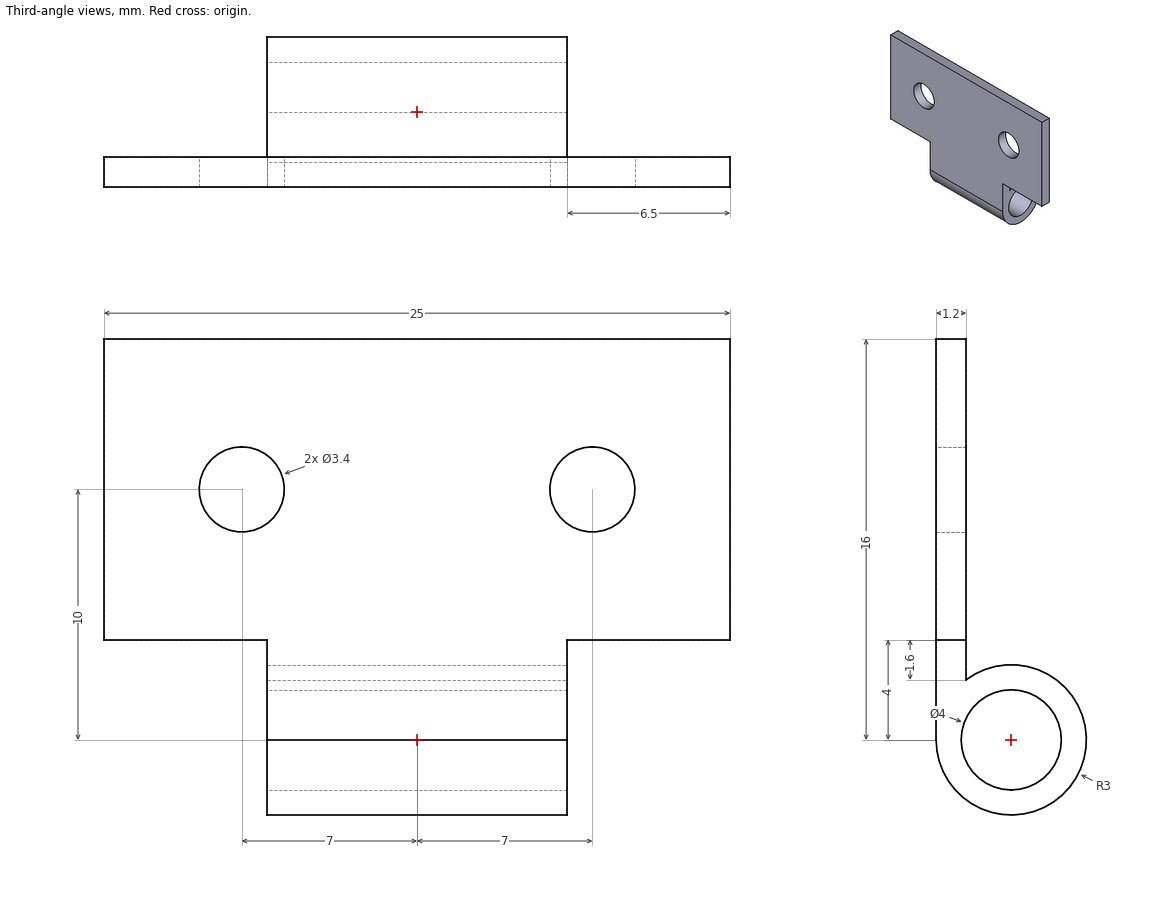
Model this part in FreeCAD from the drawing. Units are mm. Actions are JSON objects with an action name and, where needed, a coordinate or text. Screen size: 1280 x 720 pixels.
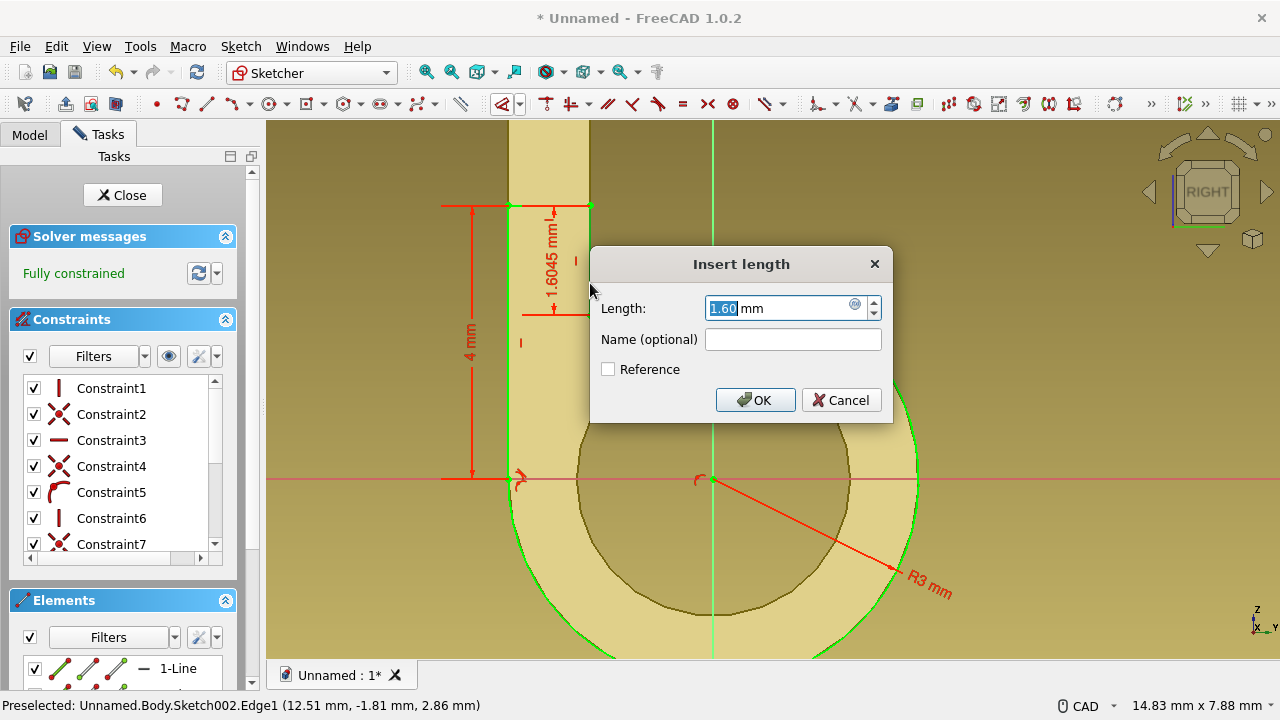
{"action": "type", "text": "1.6"}
{"action": "key", "text": "Return"}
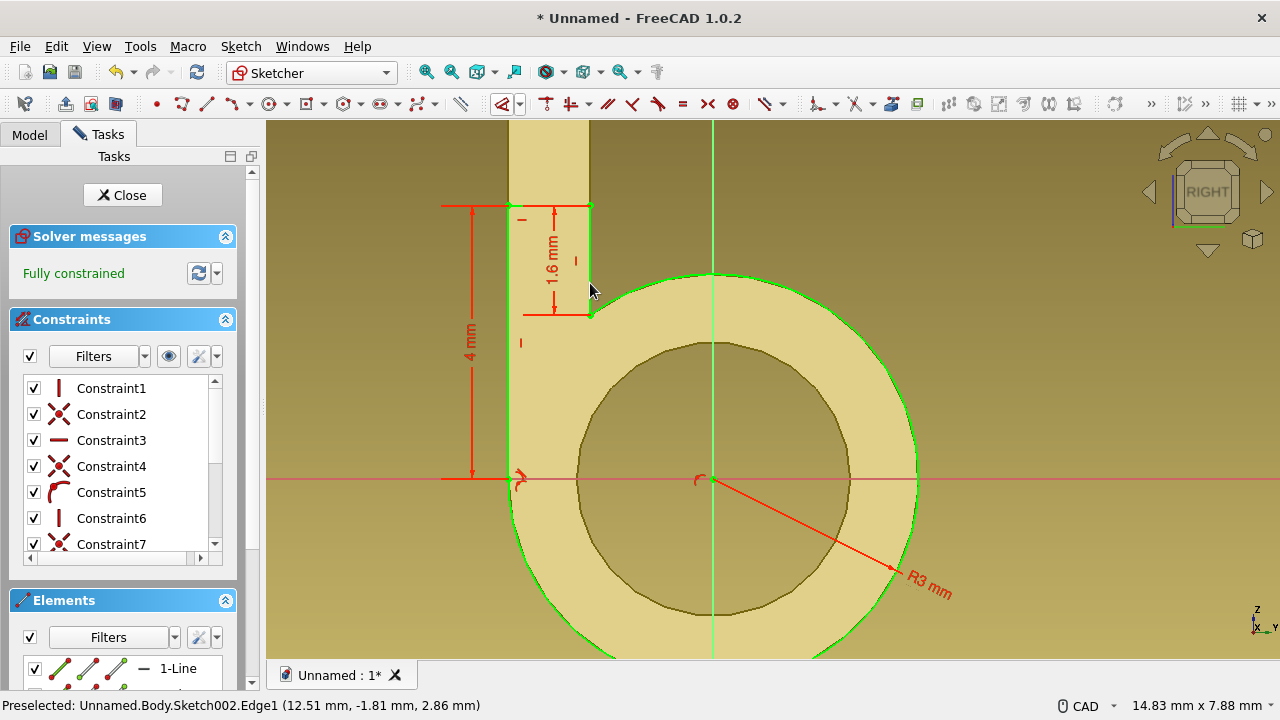
{"action": "left_click", "coordinate": [123, 195]}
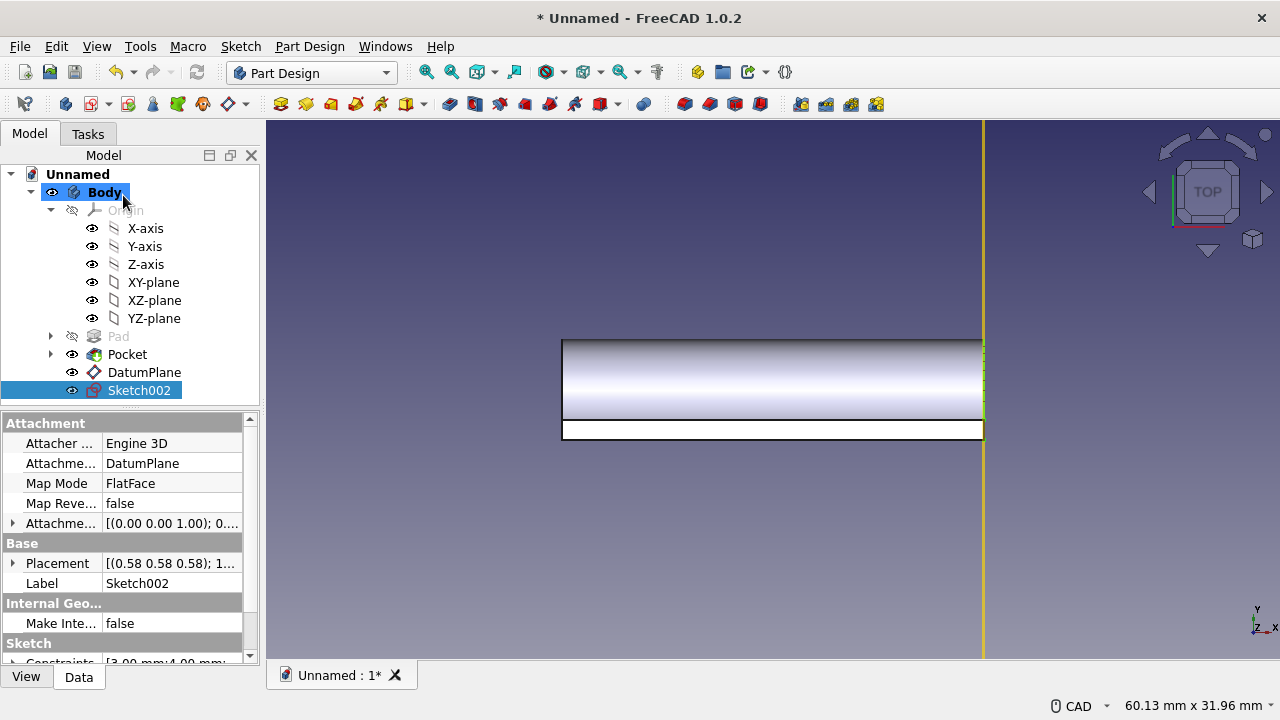
{"action": "left_click", "coordinate": [450, 104]}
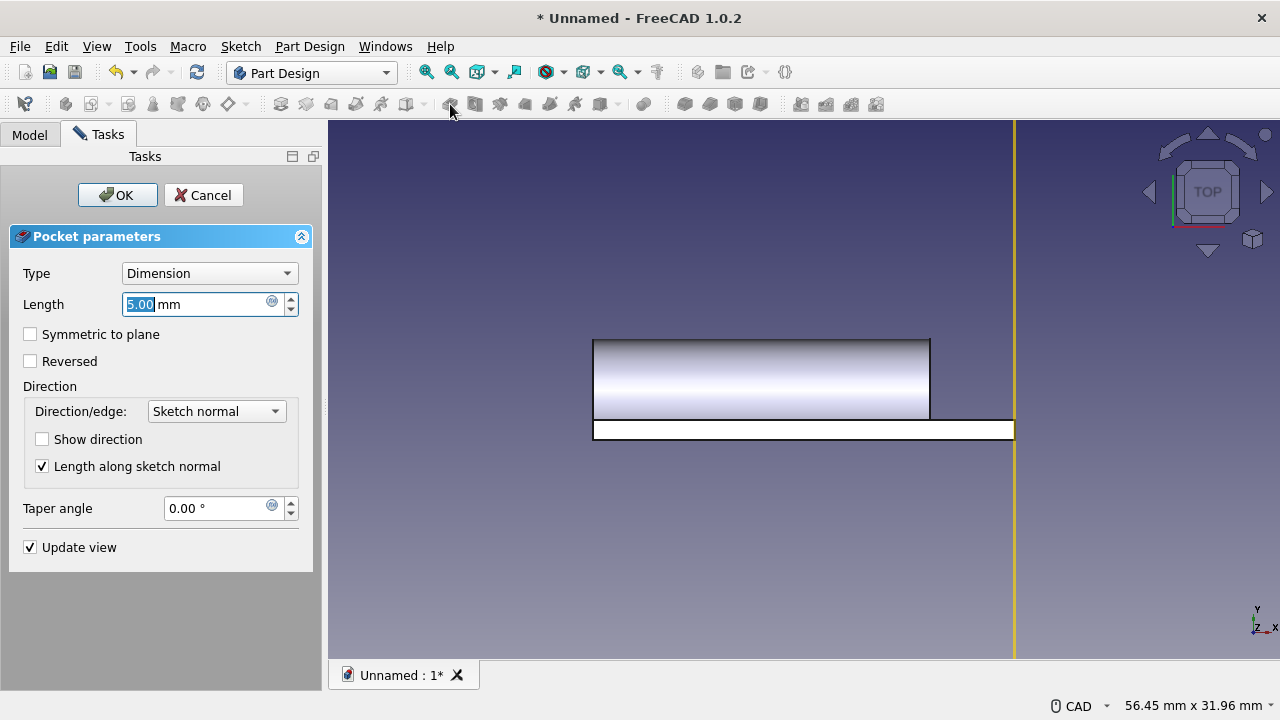
{"action": "type", "text": "6.5"}
{"action": "key", "text": "Tab"}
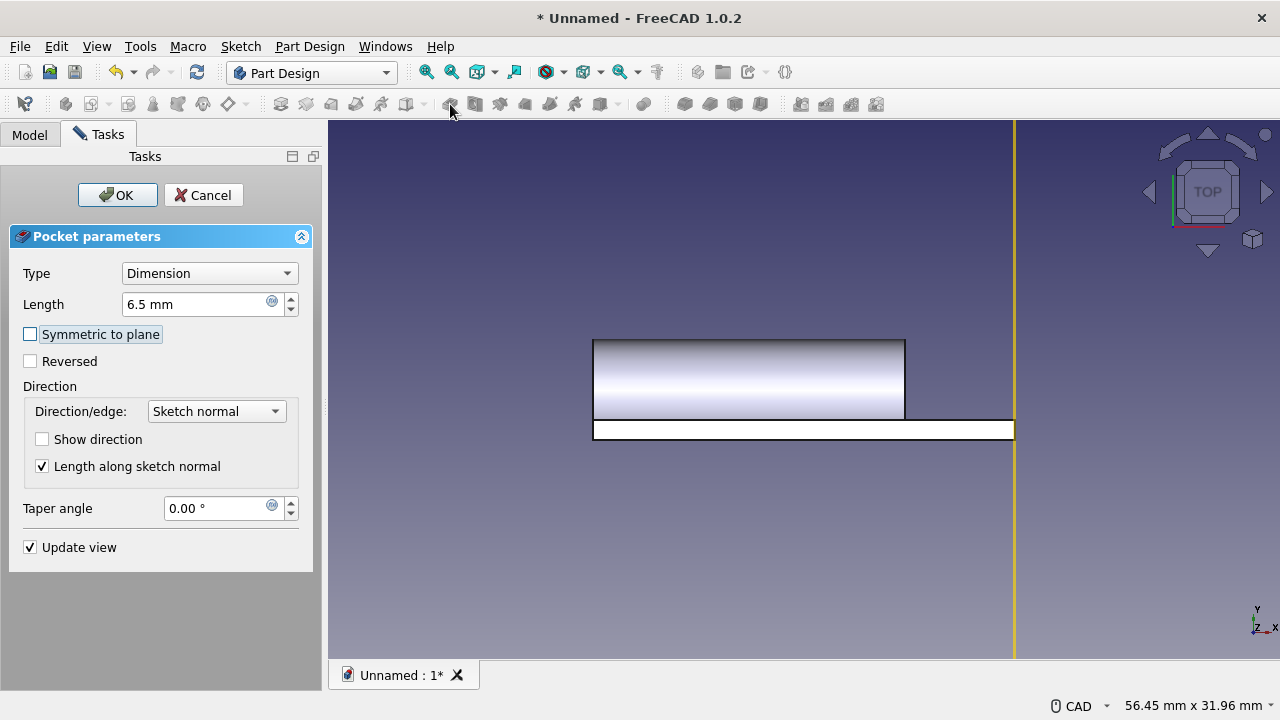
{"action": "left_click", "coordinate": [118, 195]}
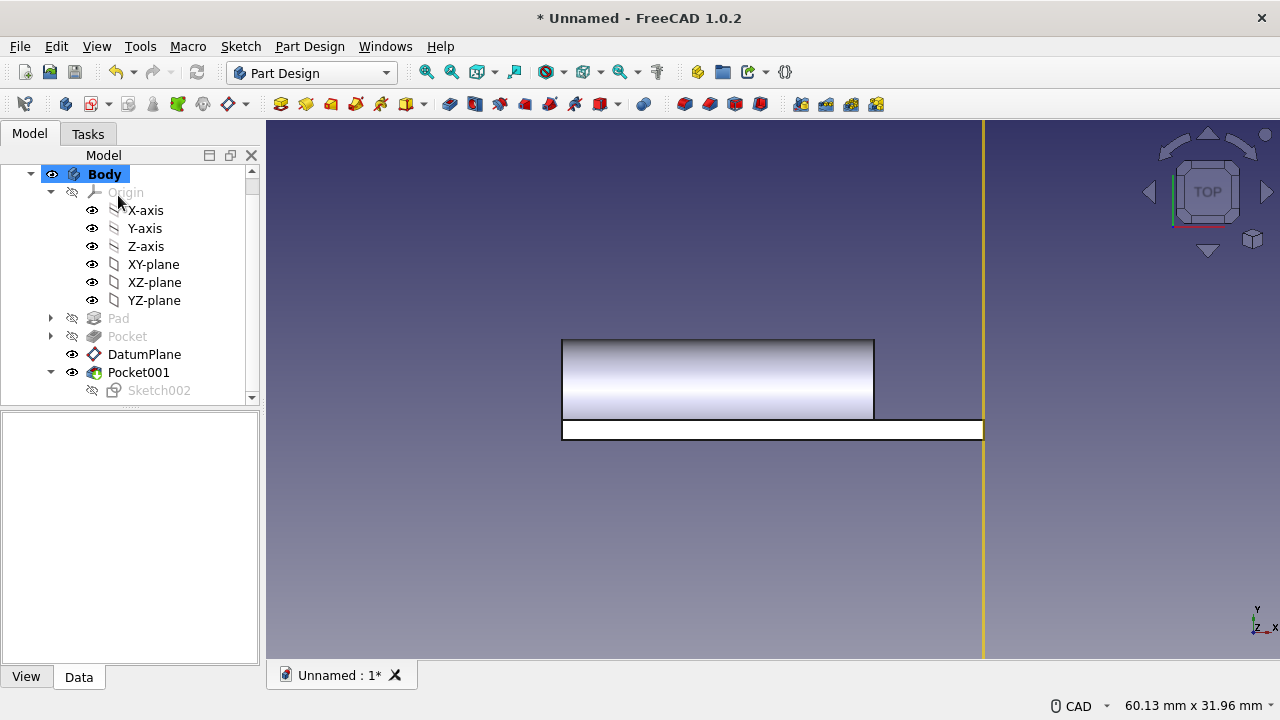
{"action": "left_click", "coordinate": [117, 354]}
{"action": "key", "text": "space"}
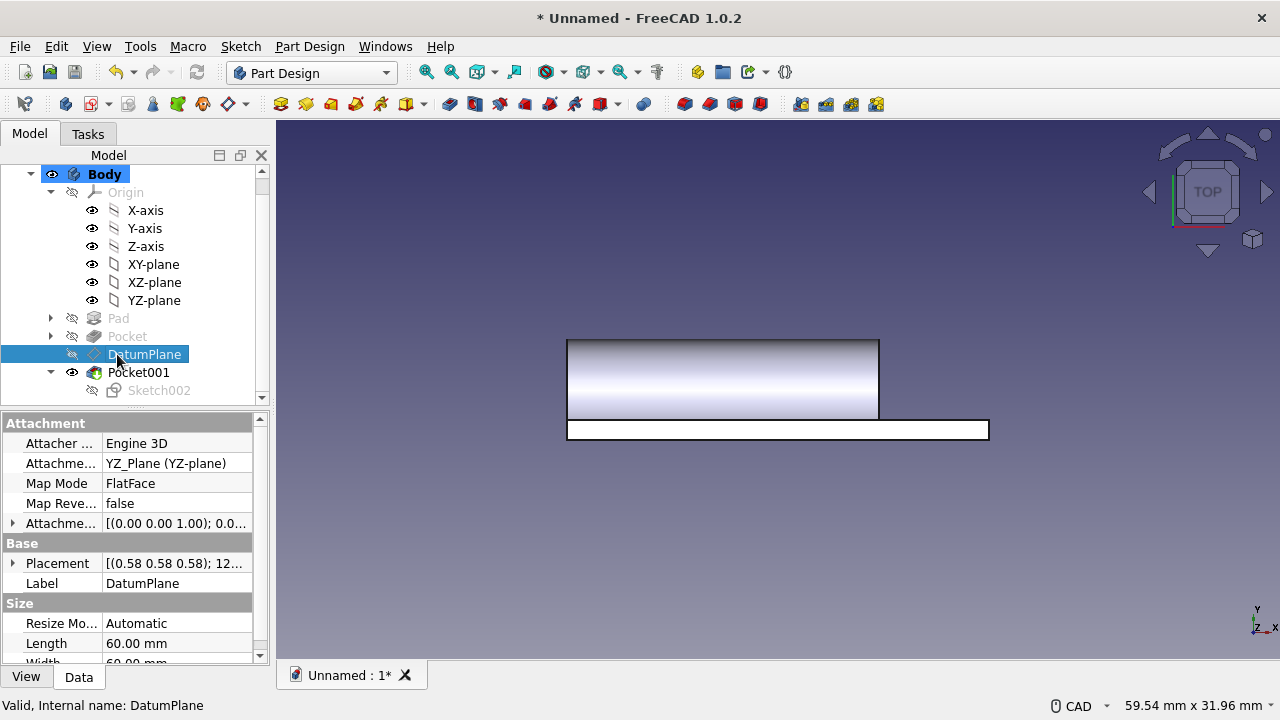
{"action": "left_click", "coordinate": [427, 72]}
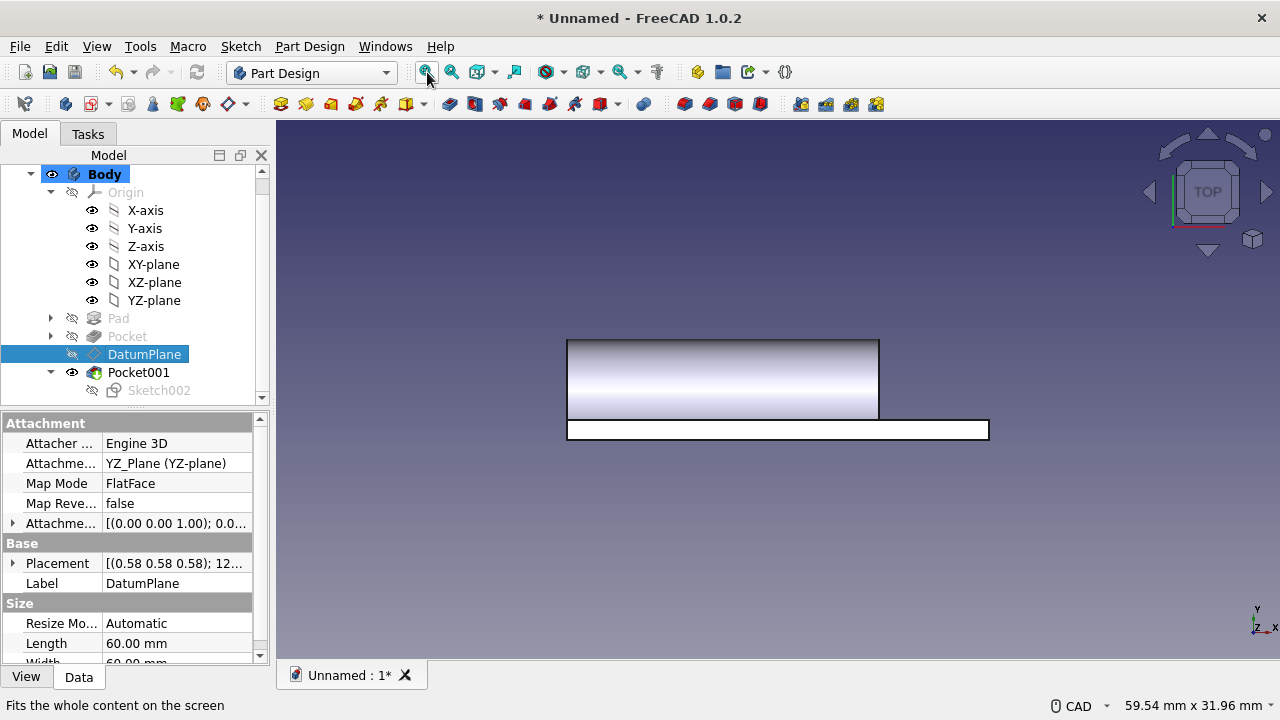
{"action": "left_click", "coordinate": [117, 372]}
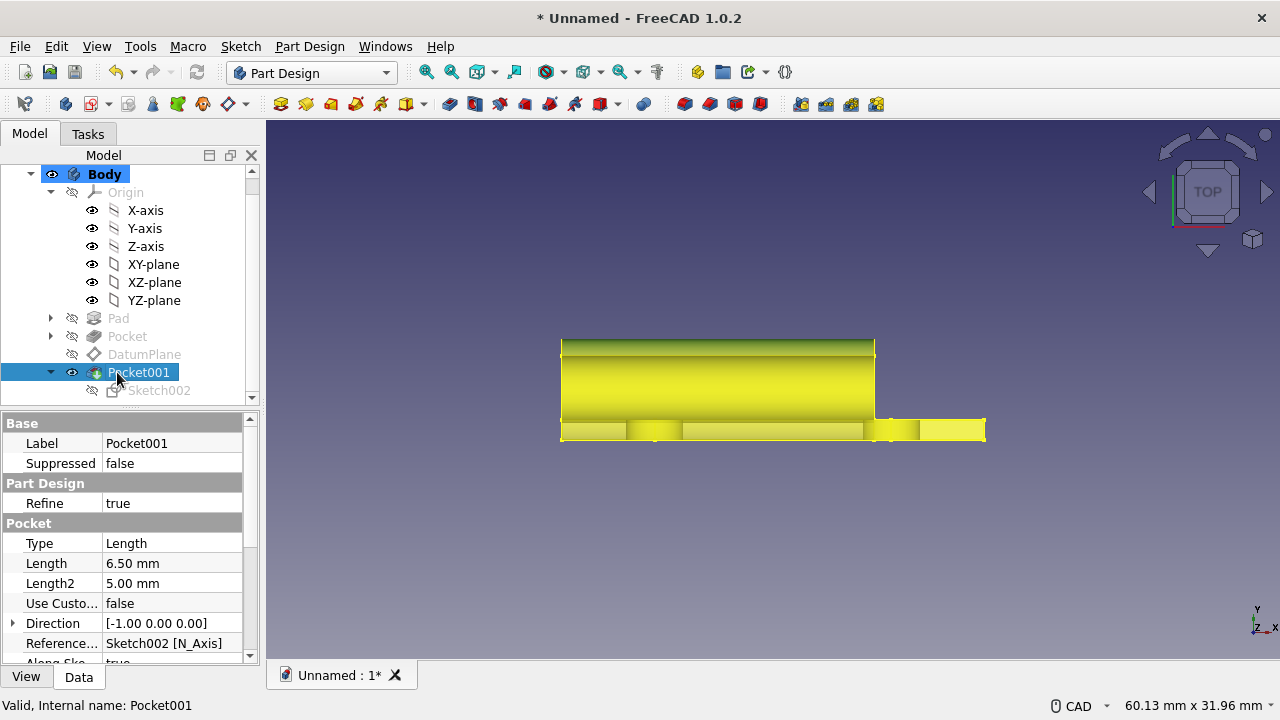
{"action": "left_click", "coordinate": [801, 104]}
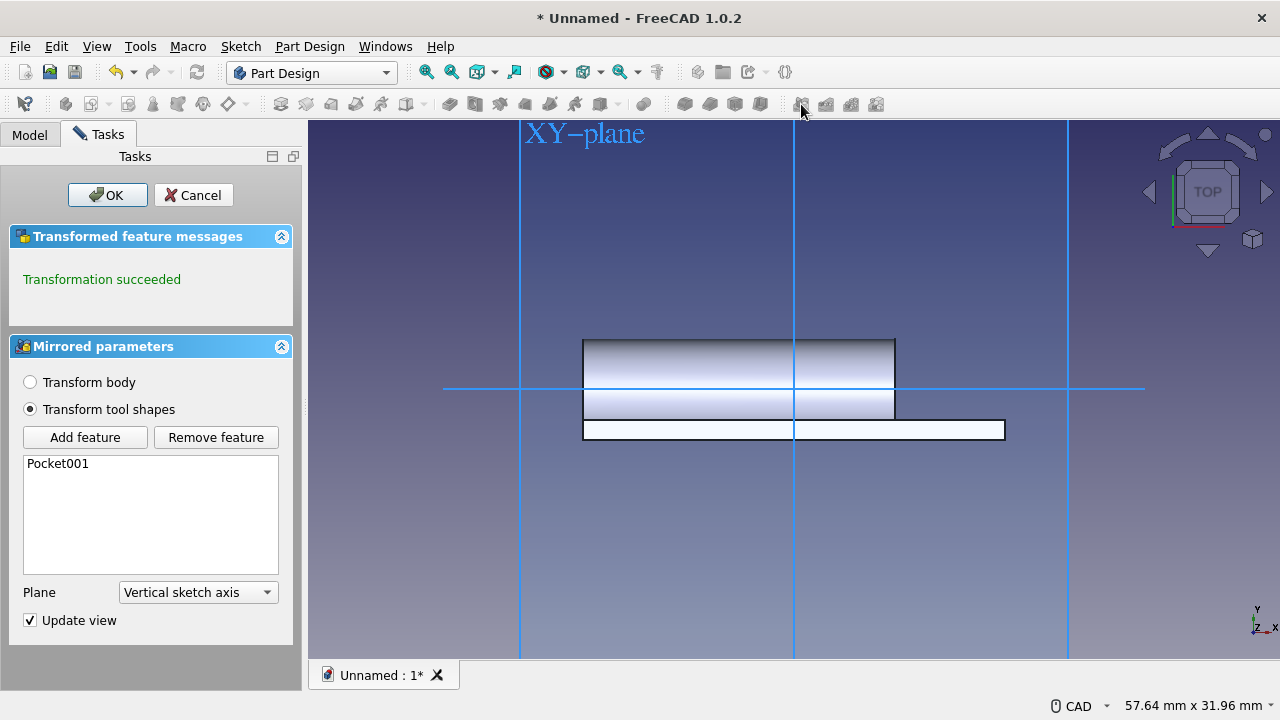
{"action": "left_click", "coordinate": [199, 592]}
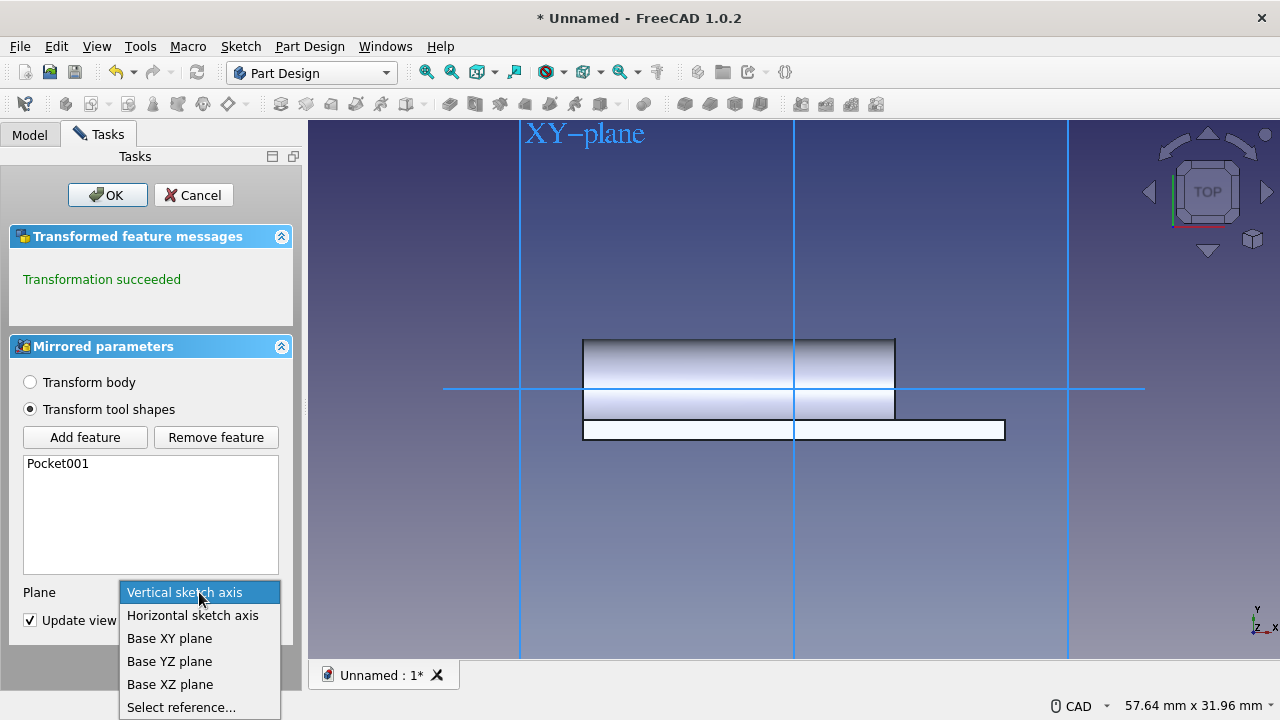
{"action": "left_click", "coordinate": [198, 662]}